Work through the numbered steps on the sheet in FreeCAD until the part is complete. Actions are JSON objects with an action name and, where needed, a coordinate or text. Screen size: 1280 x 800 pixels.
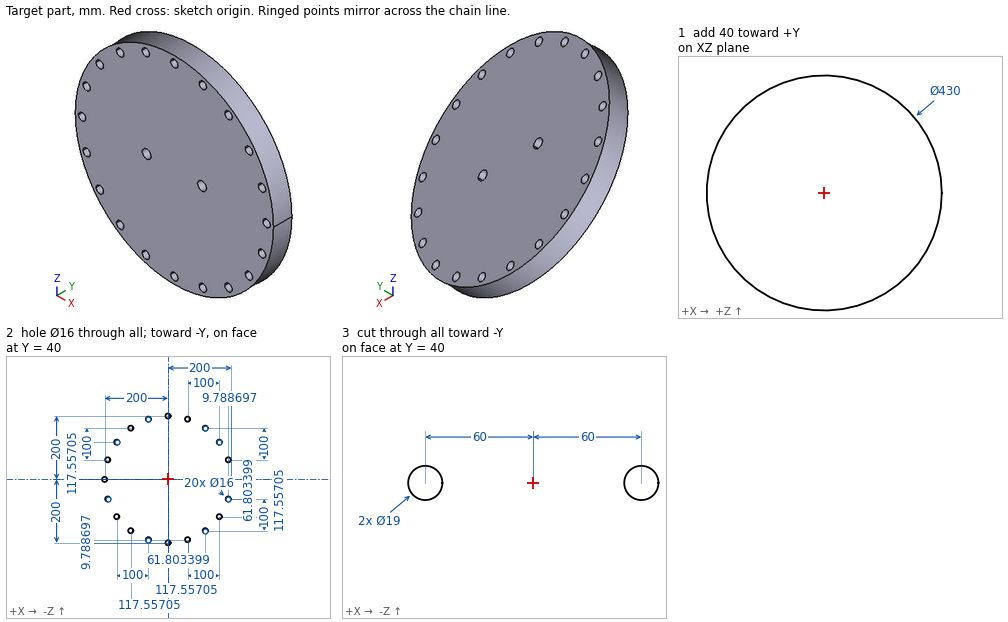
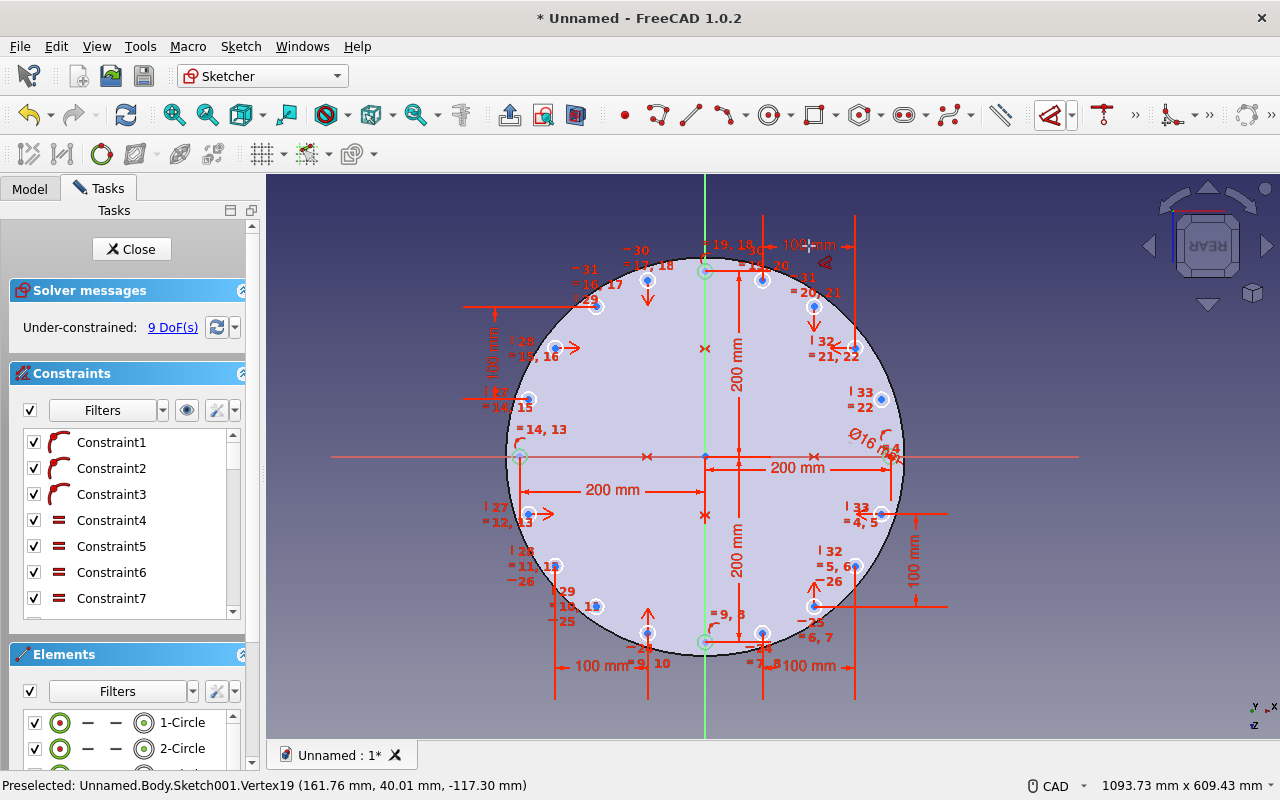
{"action": "left_click", "coordinate": [814, 307]}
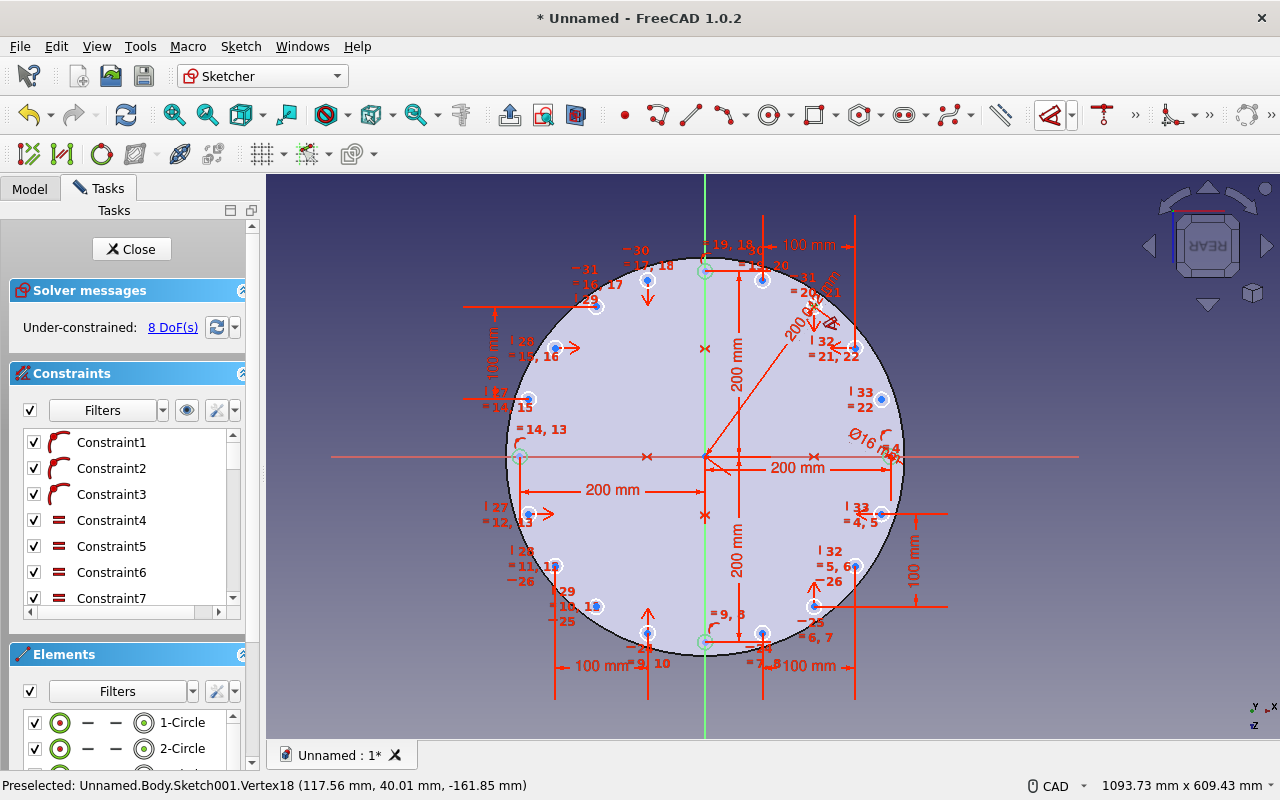
{"action": "left_click", "coordinate": [882, 400]}
{"action": "left_click", "coordinate": [916, 353]}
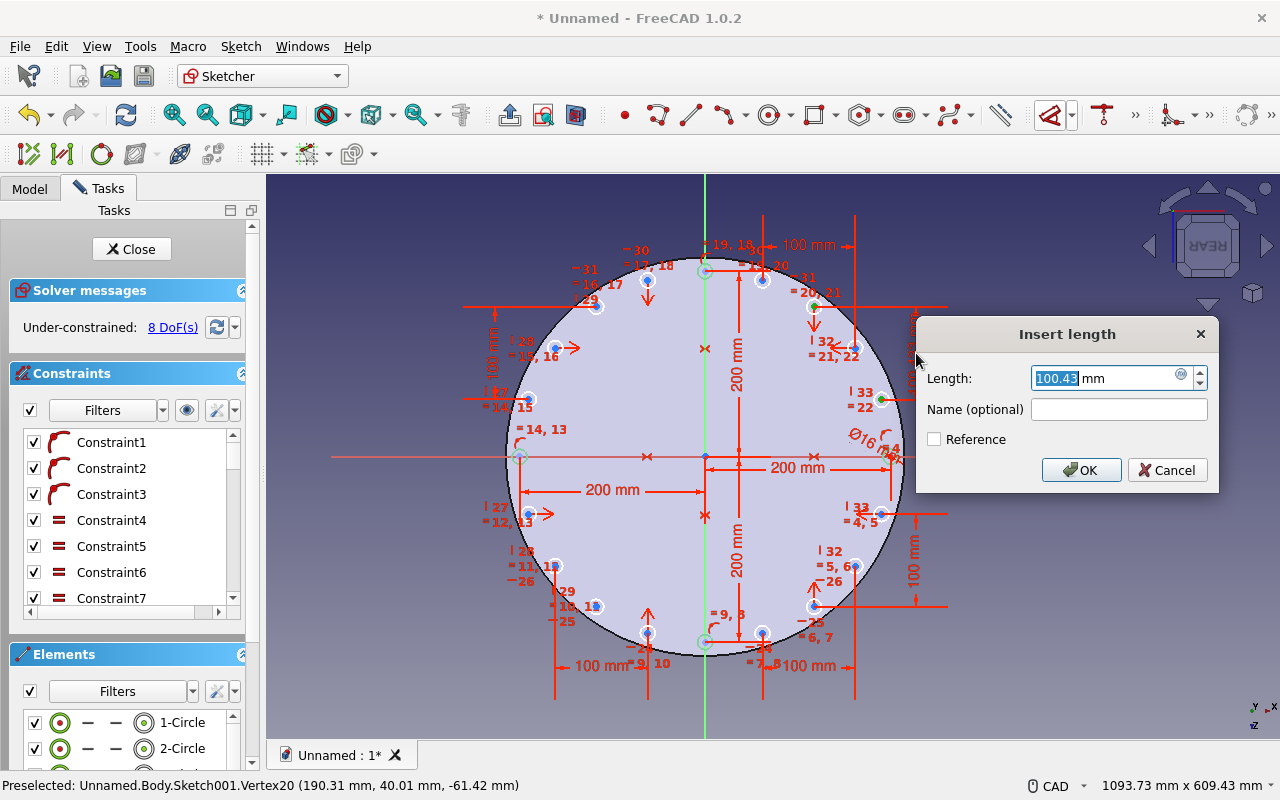
{"action": "type", "text": "100"}
{"action": "key", "text": "Return"}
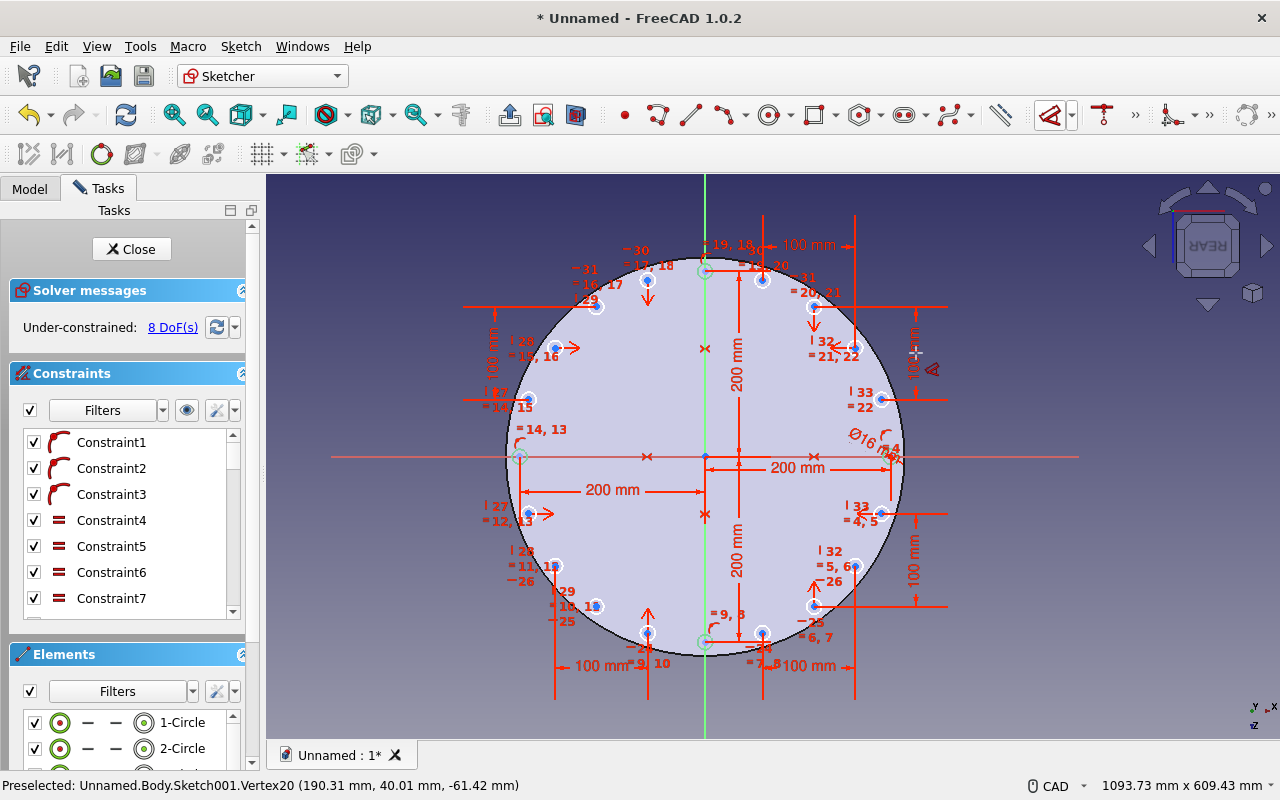
{"action": "left_click", "coordinate": [882, 514]}
{"action": "left_click", "coordinate": [916, 485]}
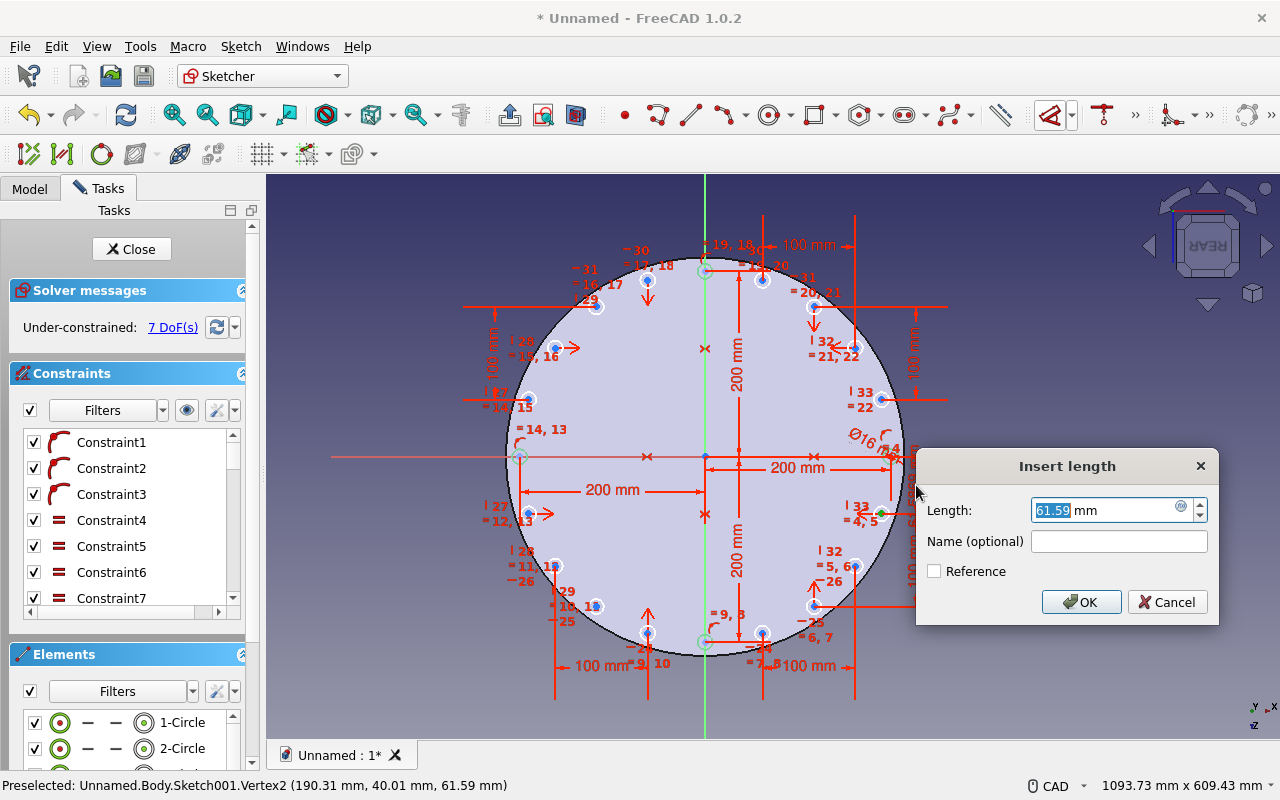
{"action": "type", "text": "61.803399"}
{"action": "key", "text": "Return"}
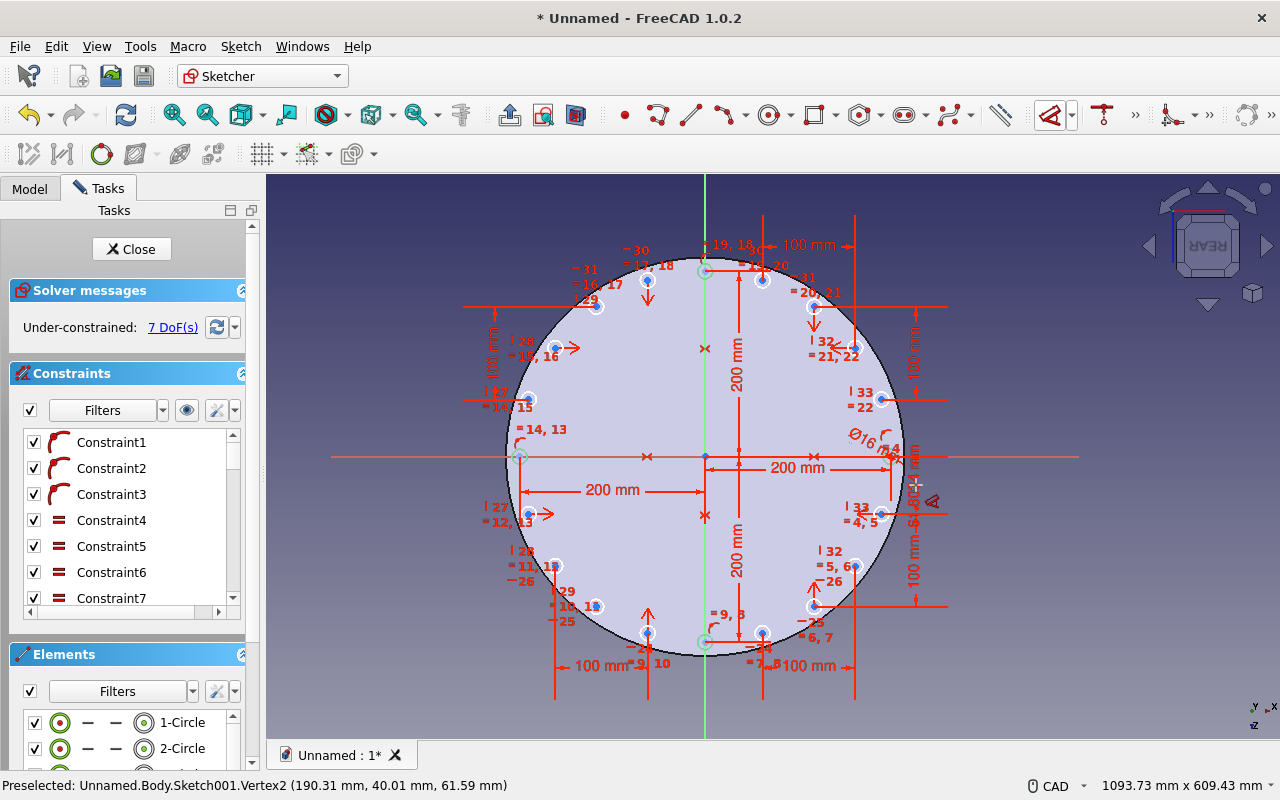
{"action": "left_click", "coordinate": [855, 566]}
{"action": "left_click", "coordinate": [889, 537]}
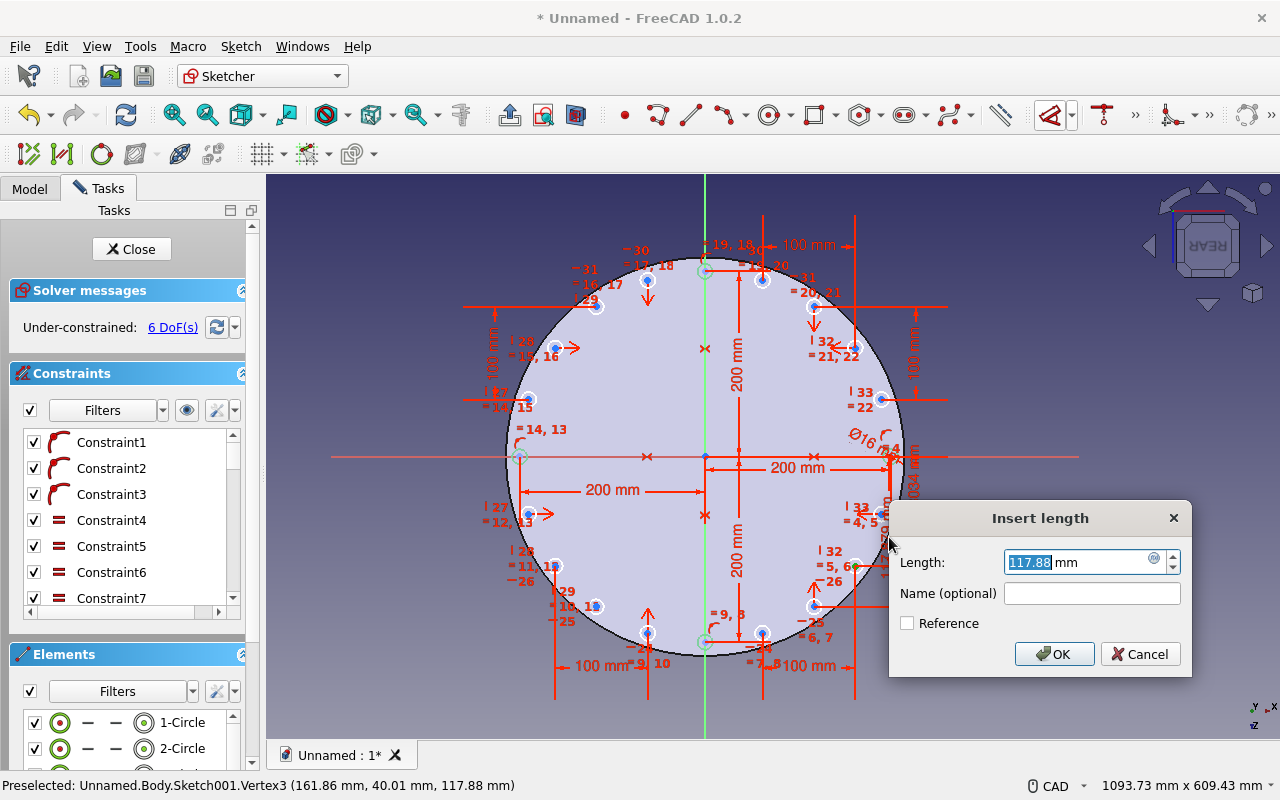
{"action": "type", "text": "117.55705"}
{"action": "key", "text": "Return"}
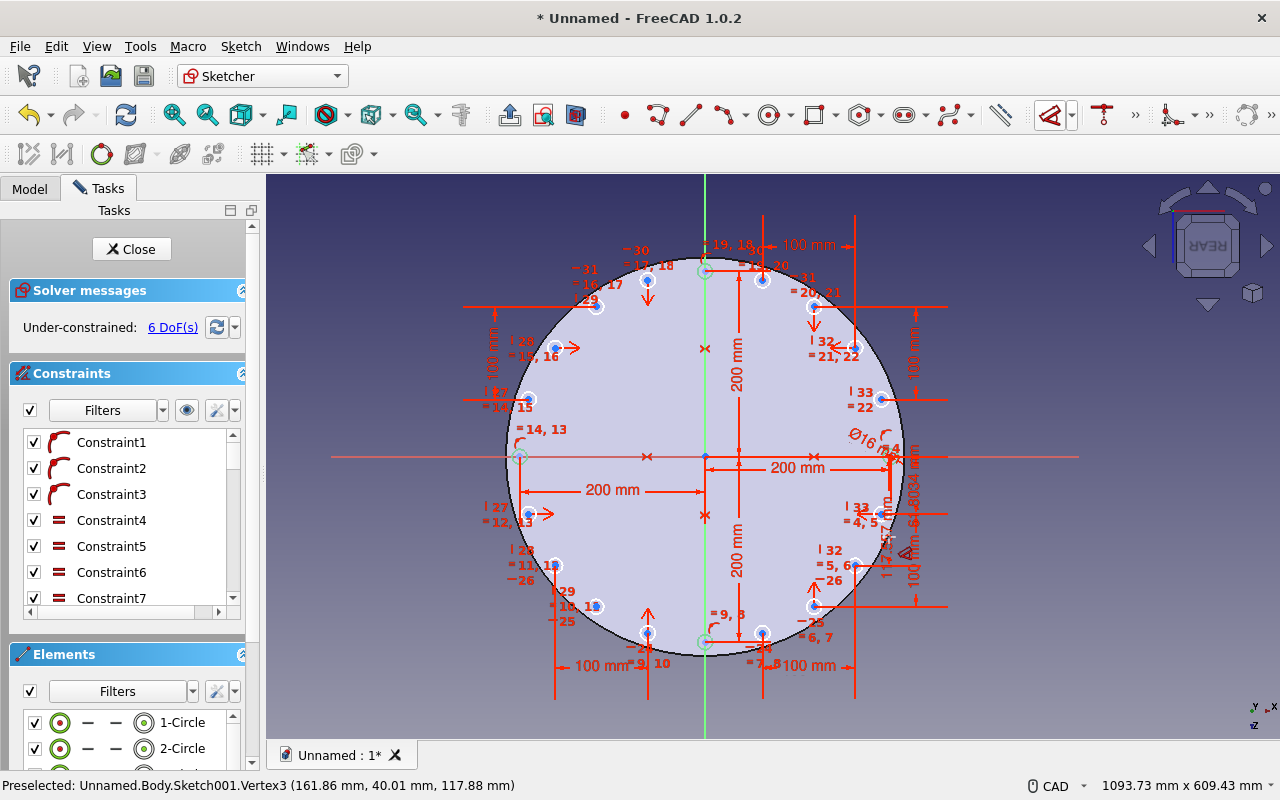
{"action": "left_click", "coordinate": [814, 607]}
{"action": "left_click", "coordinate": [735, 641]}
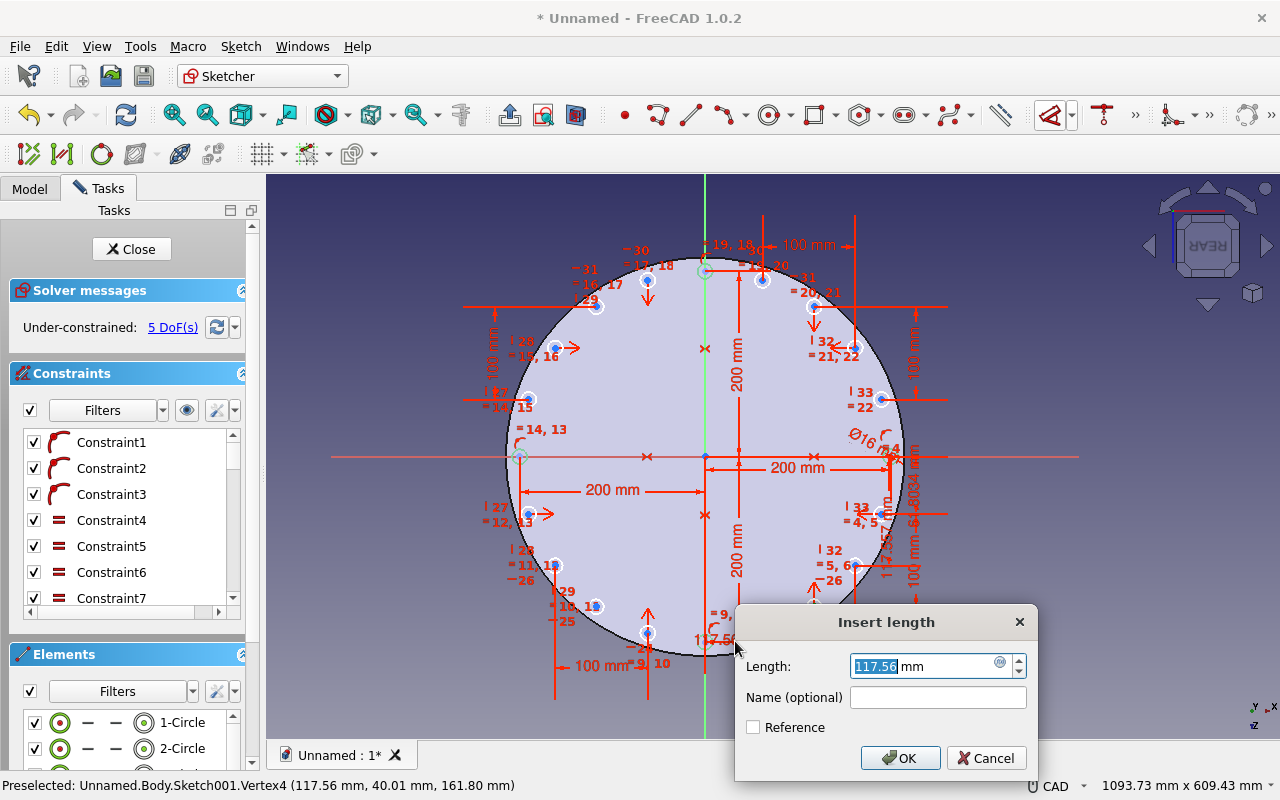
{"action": "type", "text": "117.55705"}
{"action": "key", "text": "Return"}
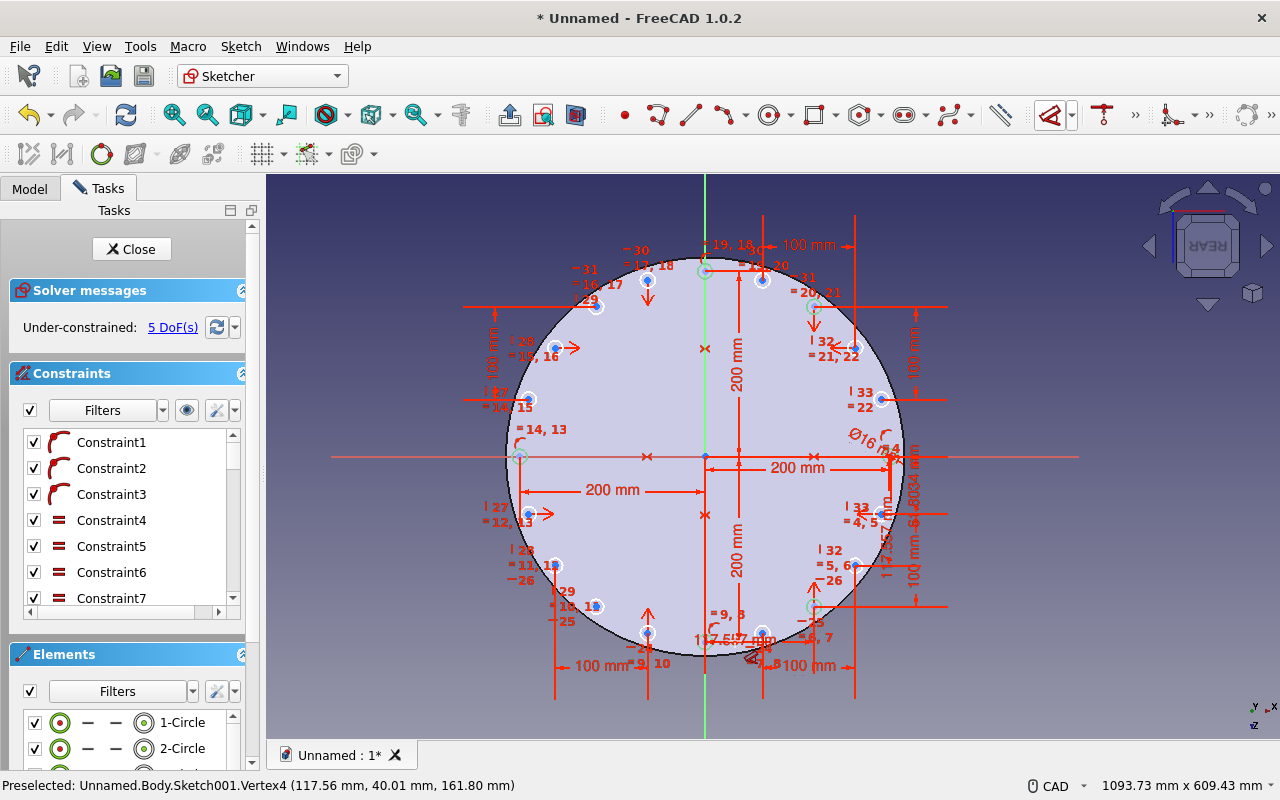
{"action": "left_click", "coordinate": [763, 633]}
{"action": "left_click", "coordinate": [734, 667]}